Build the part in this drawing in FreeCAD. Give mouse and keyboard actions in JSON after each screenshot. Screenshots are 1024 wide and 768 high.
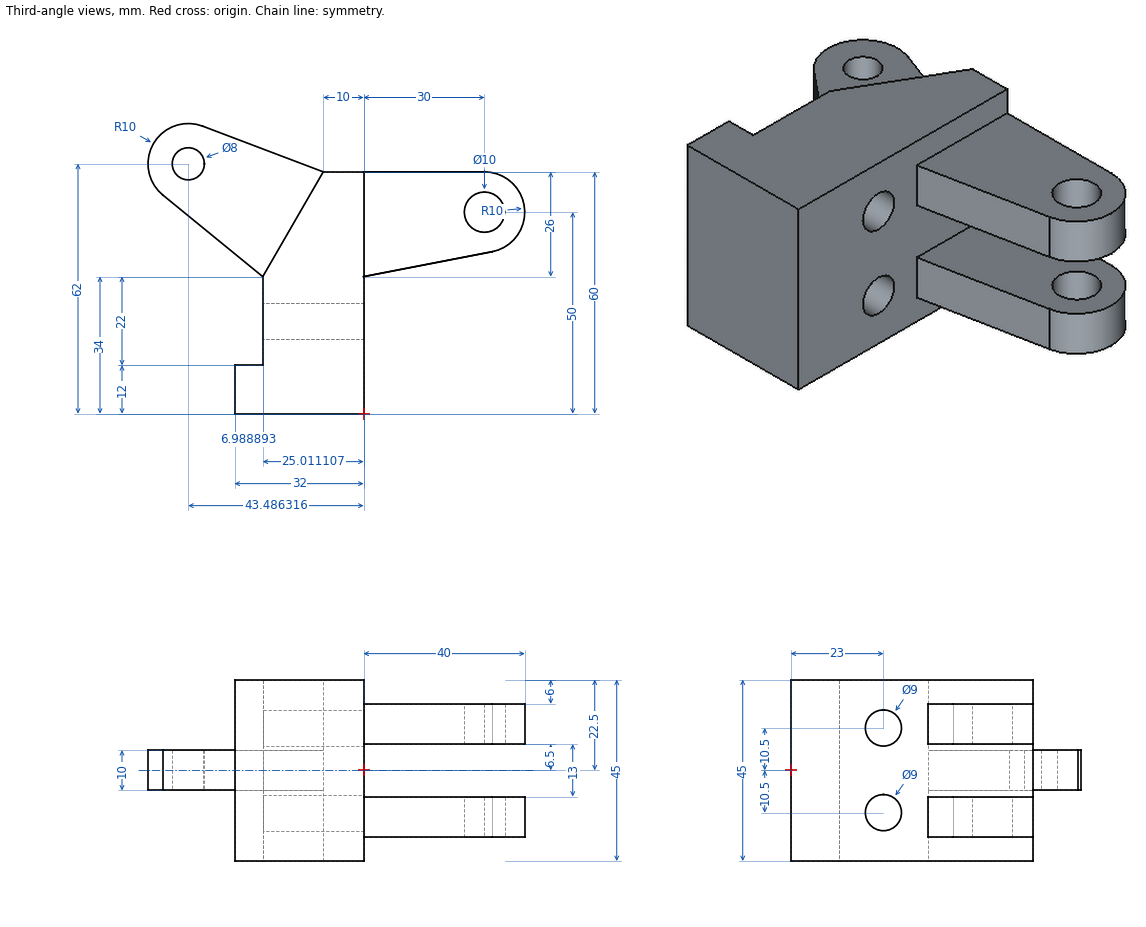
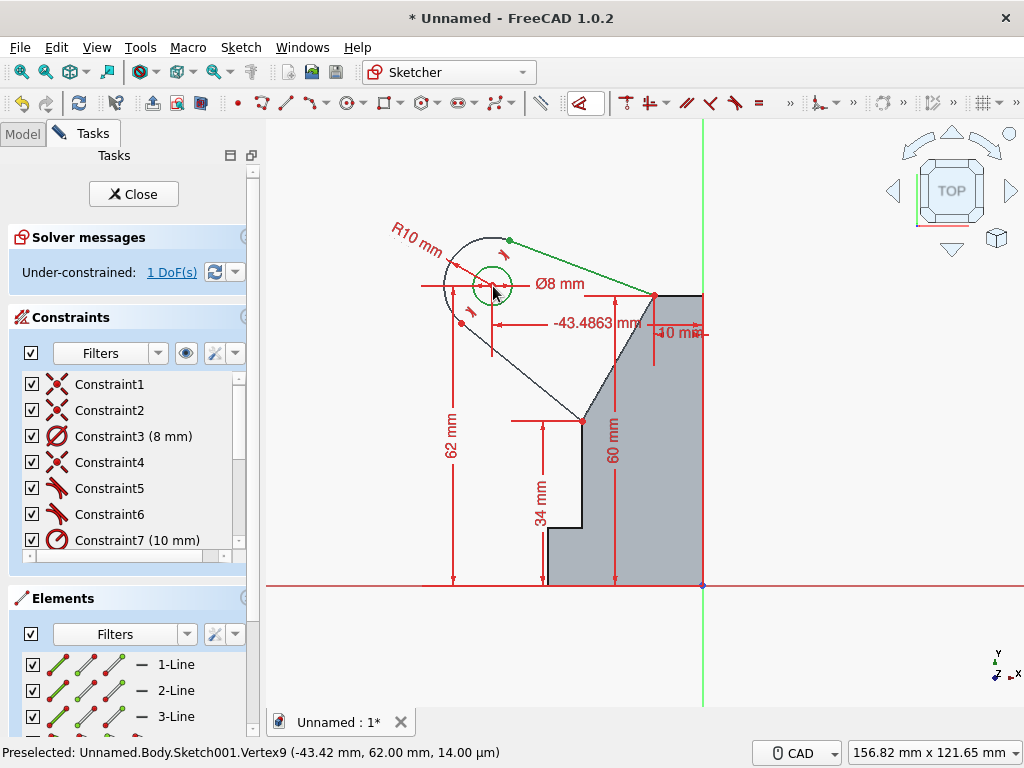
{"action": "left_click", "coordinate": [582, 421]}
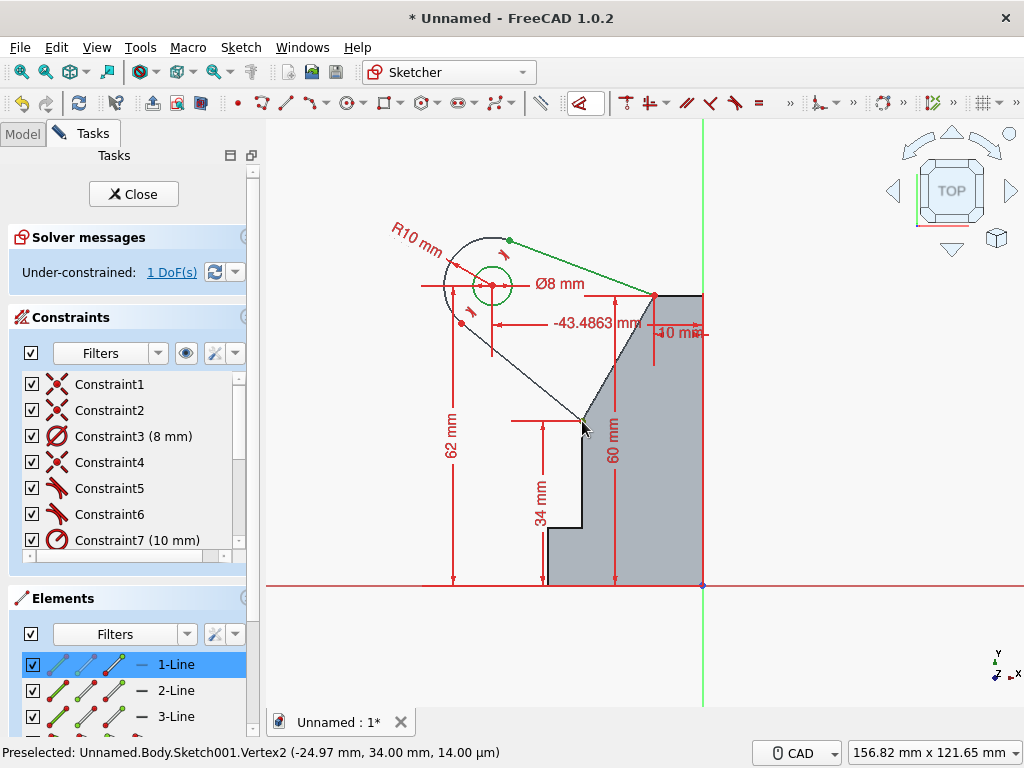
{"action": "key", "text": "l"}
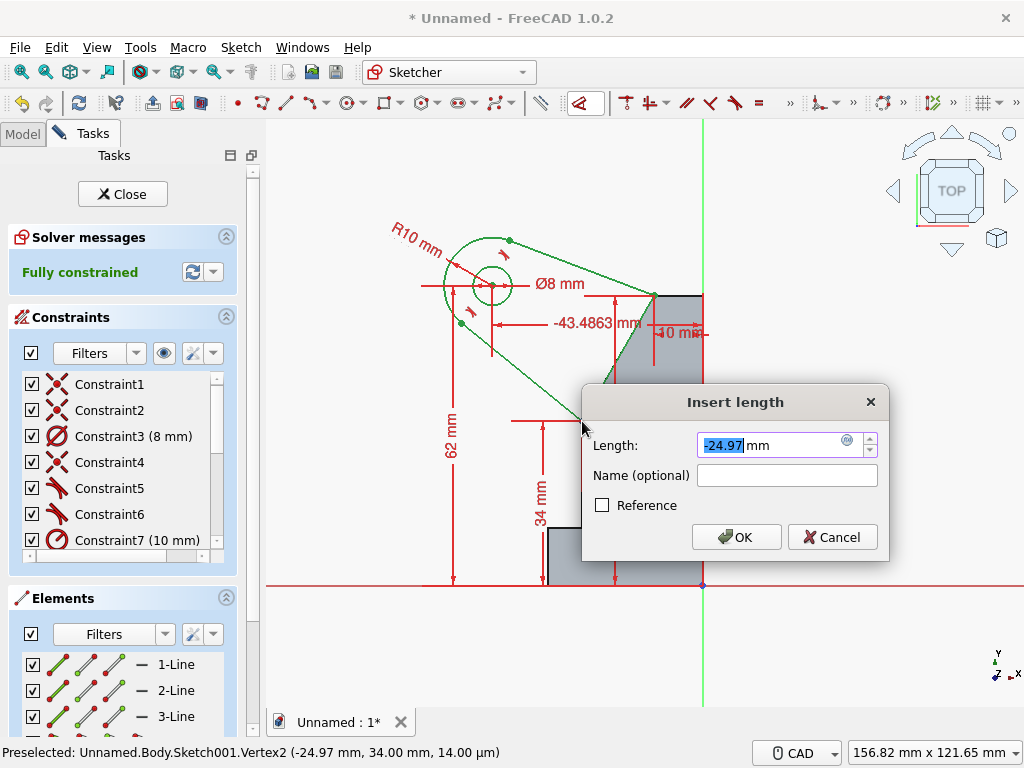
{"action": "type", "text": "-25.011107"}
{"action": "key", "text": "Return"}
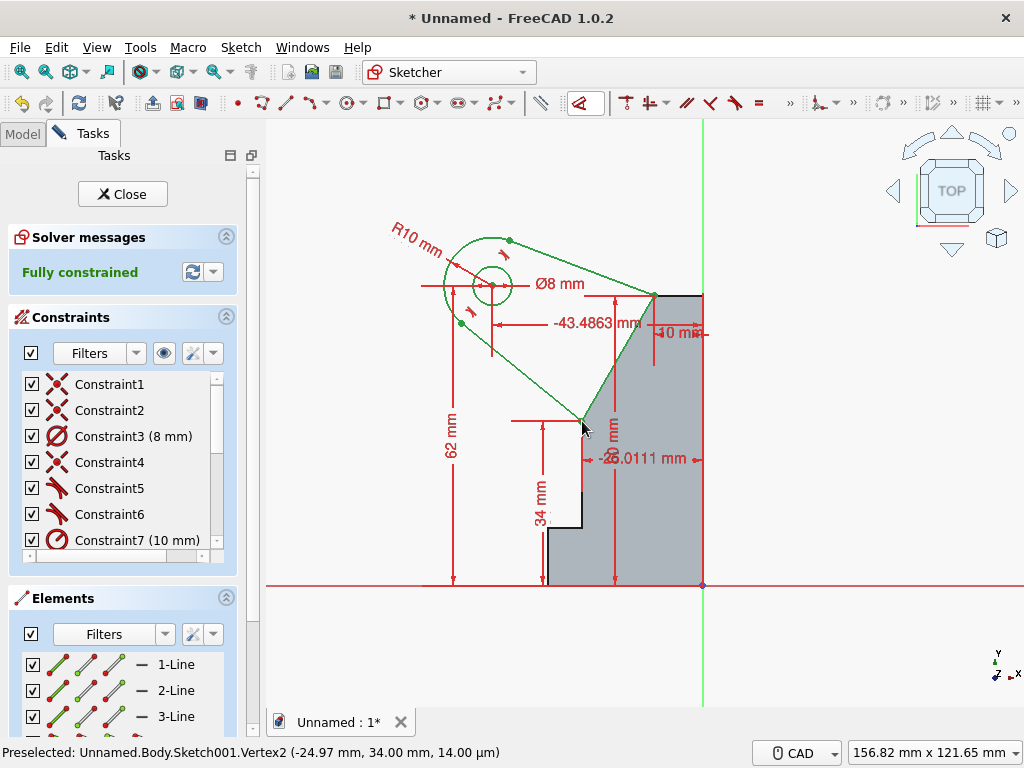
{"action": "left_click", "coordinate": [123, 194]}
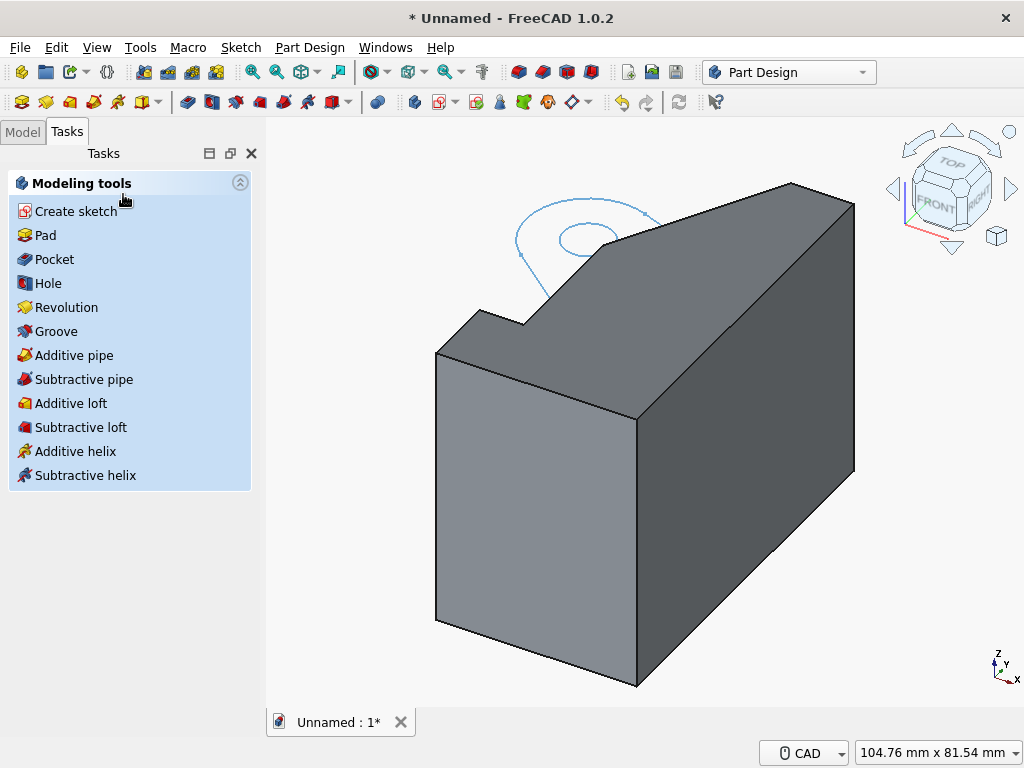
{"action": "left_click", "coordinate": [22, 102]}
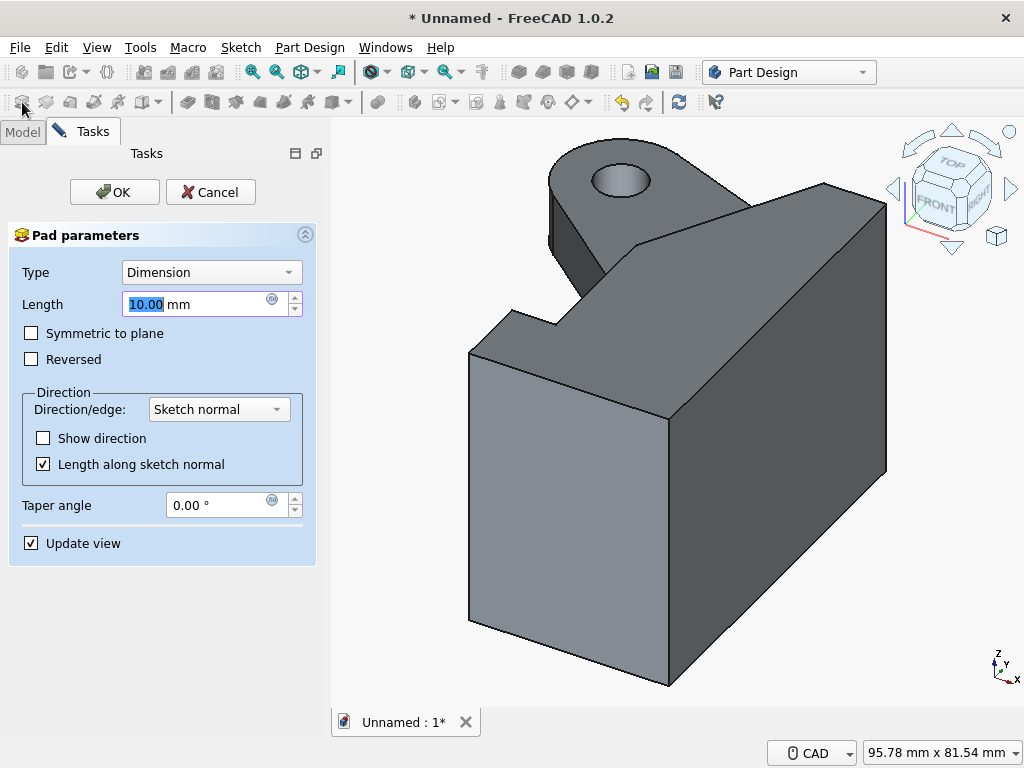
{"action": "type", "text": "10"}
{"action": "key", "text": "Tab"}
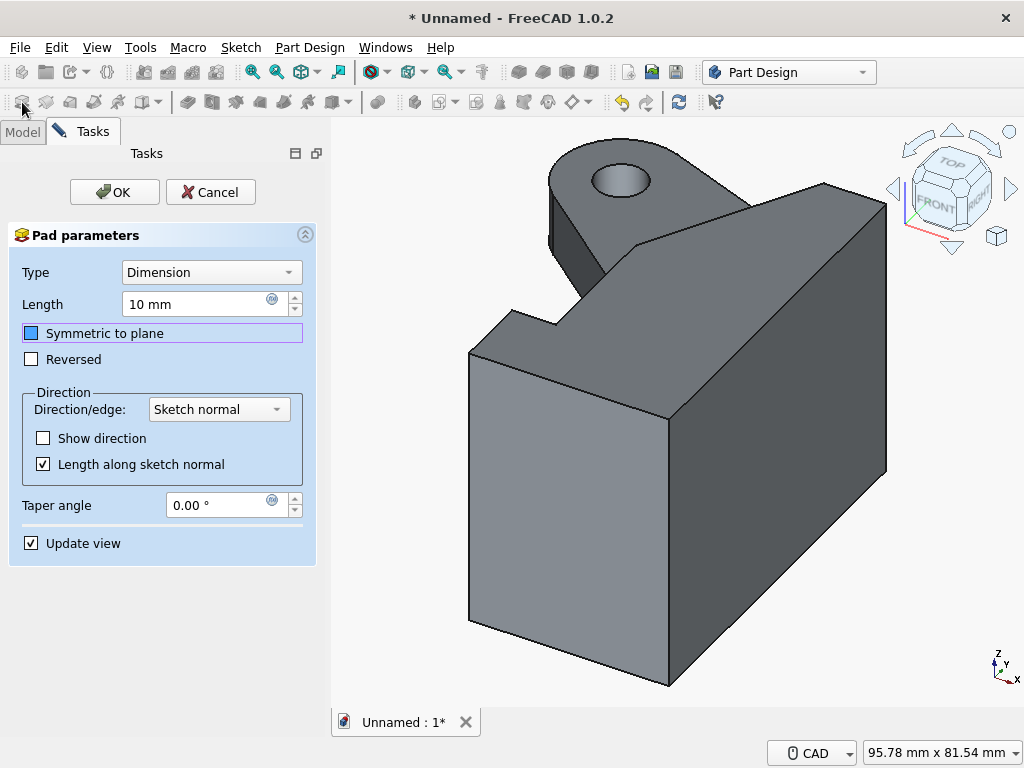
{"action": "left_click", "coordinate": [30, 333]}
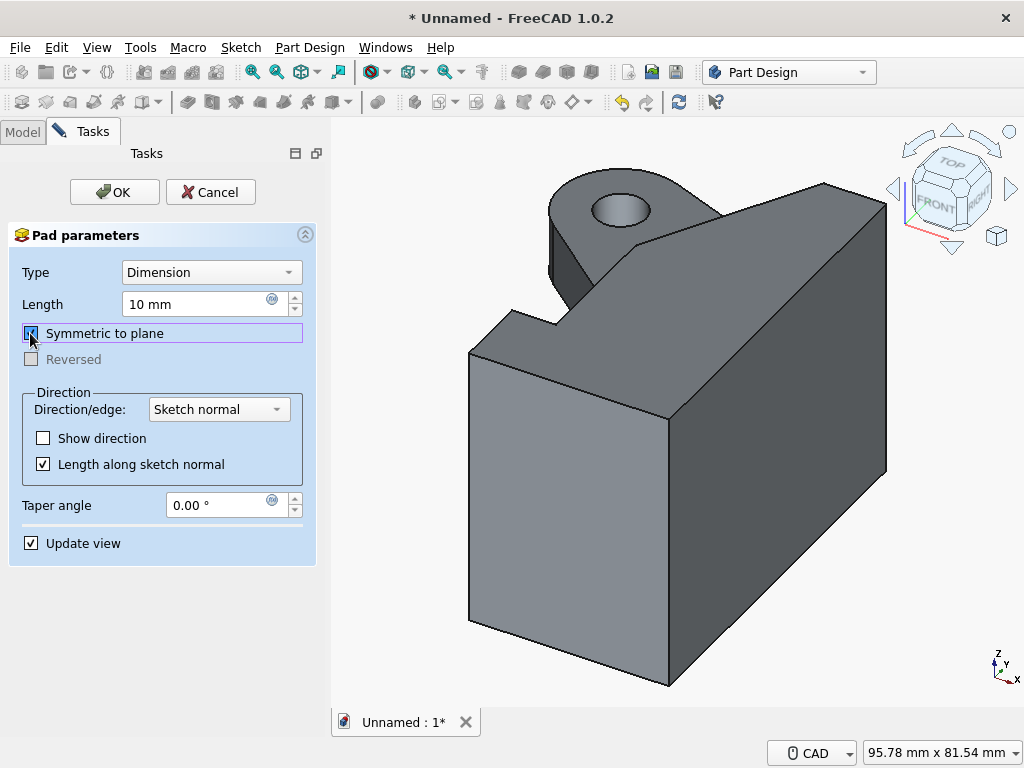
{"action": "left_click", "coordinate": [115, 192]}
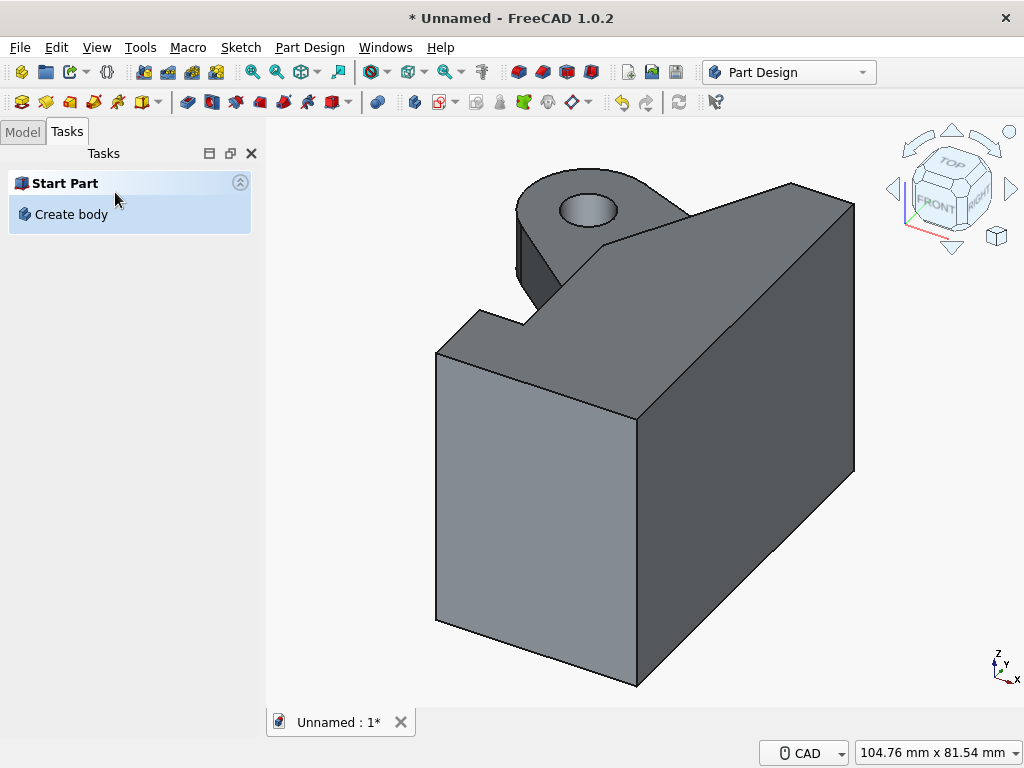
{"action": "left_click", "coordinate": [254, 72]}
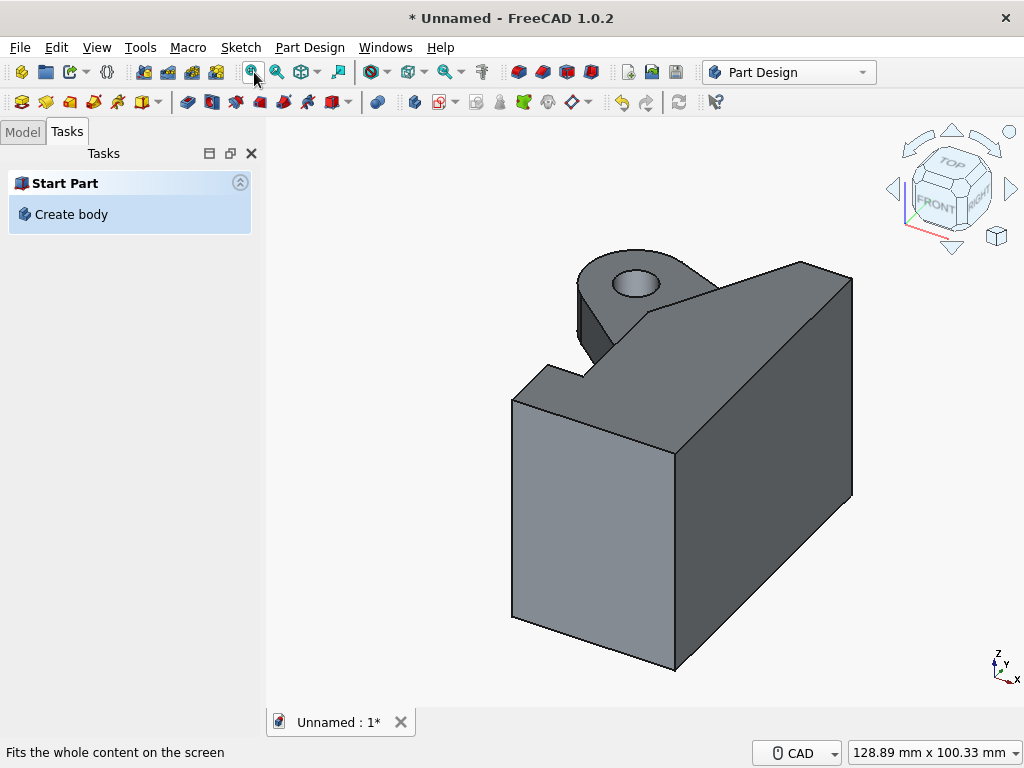
{"action": "key", "text": "6"}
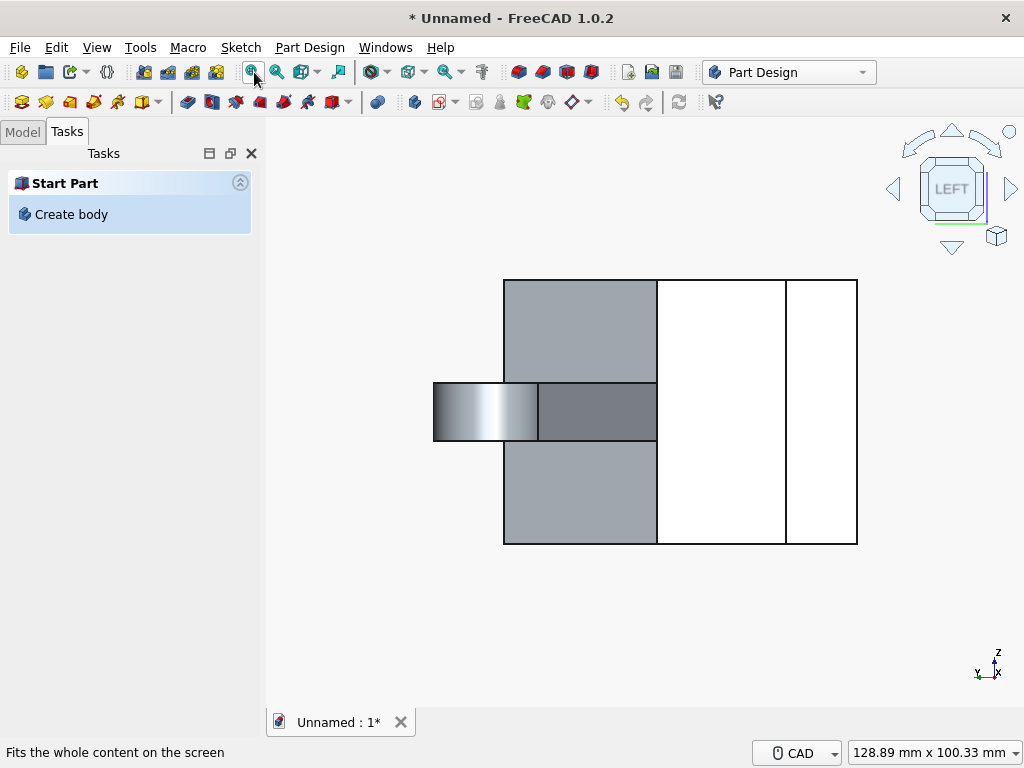
{"action": "left_click", "coordinate": [721, 373]}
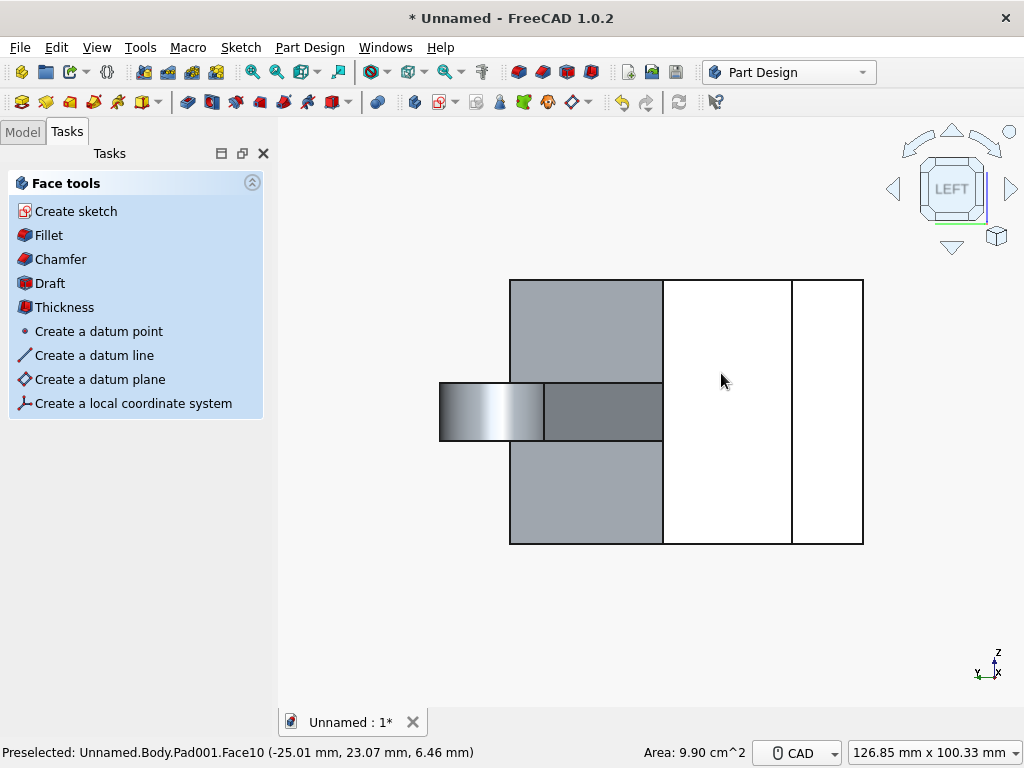
{"action": "left_click", "coordinate": [440, 102]}